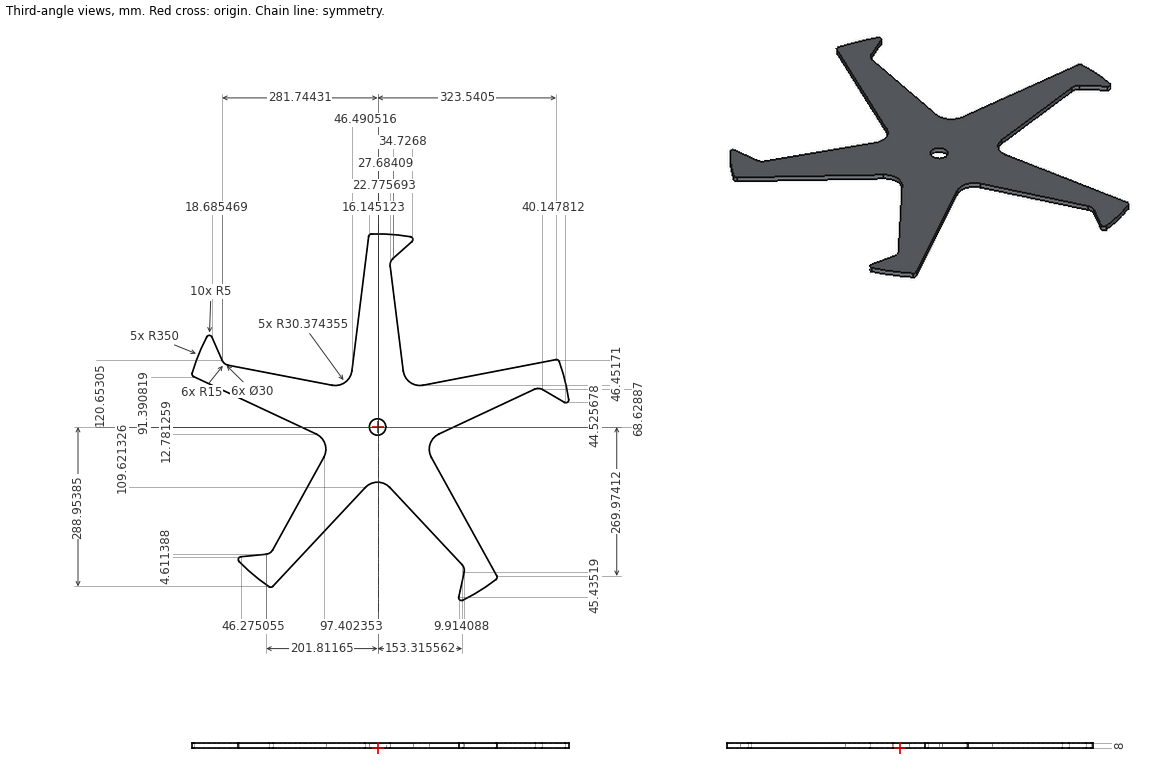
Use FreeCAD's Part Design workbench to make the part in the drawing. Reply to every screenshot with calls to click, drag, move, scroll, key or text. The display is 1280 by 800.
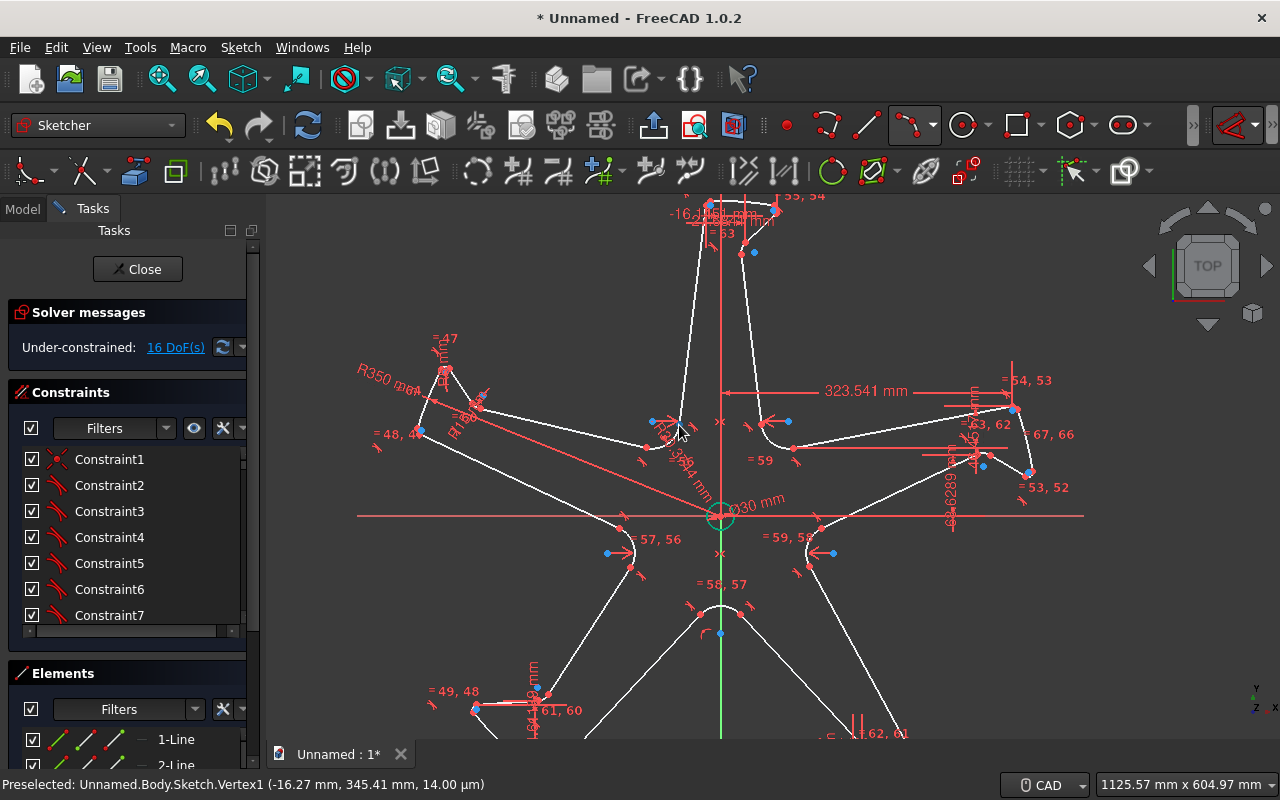
click(680, 425)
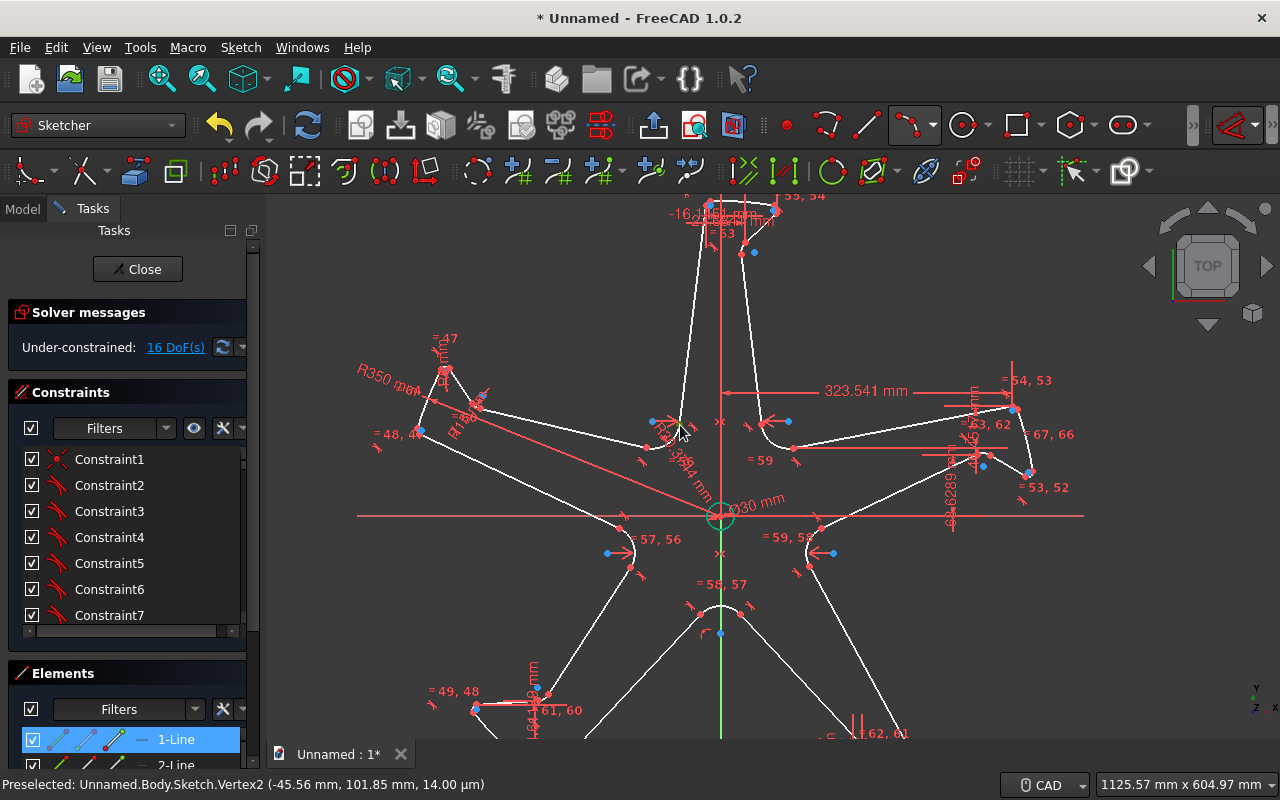
key(l)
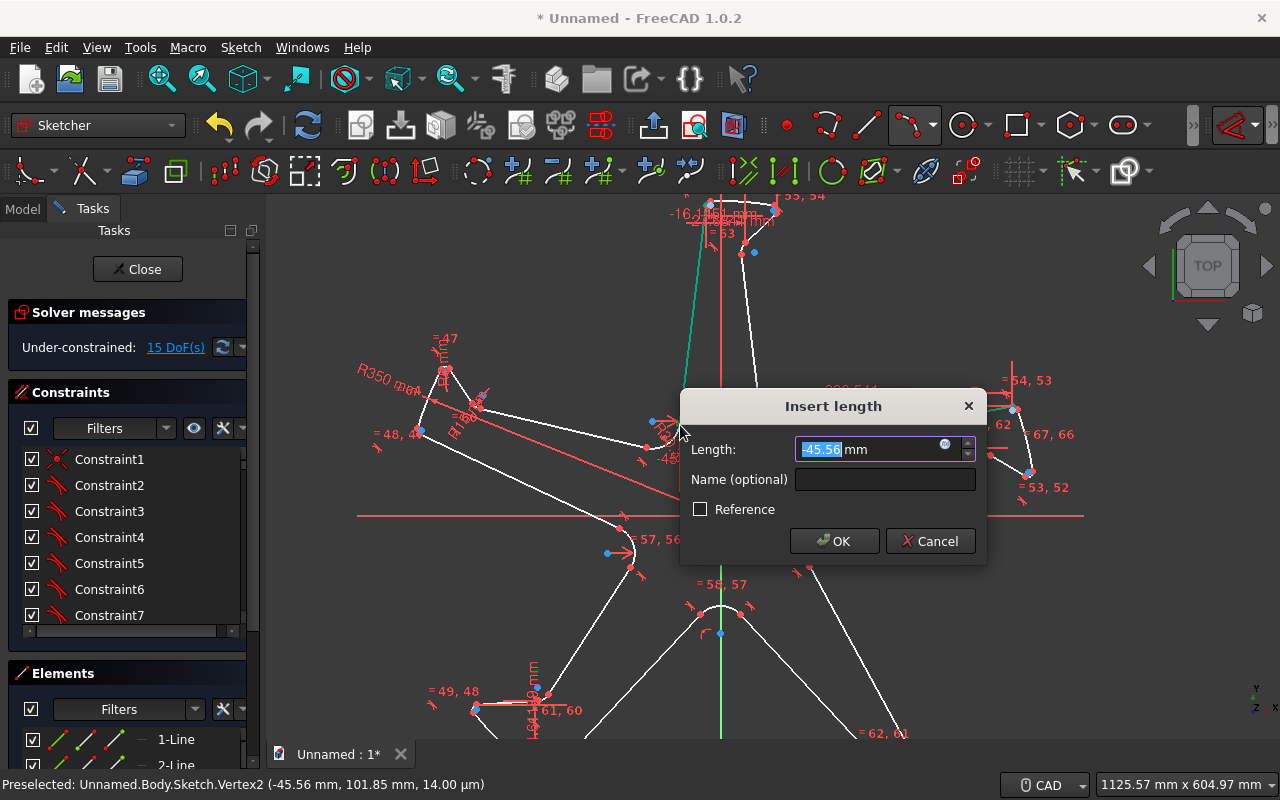
text(-46.490516)
key(Return)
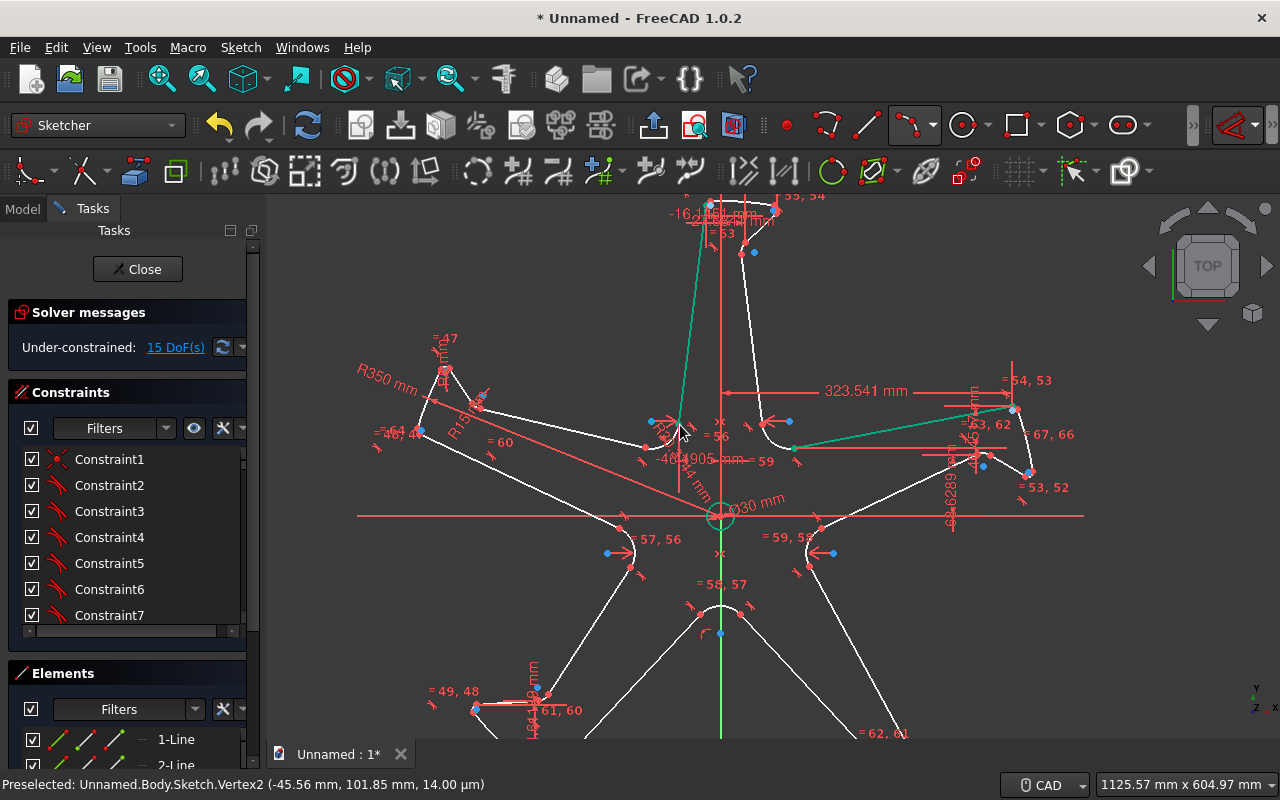
scroll(472, 403, up, 2)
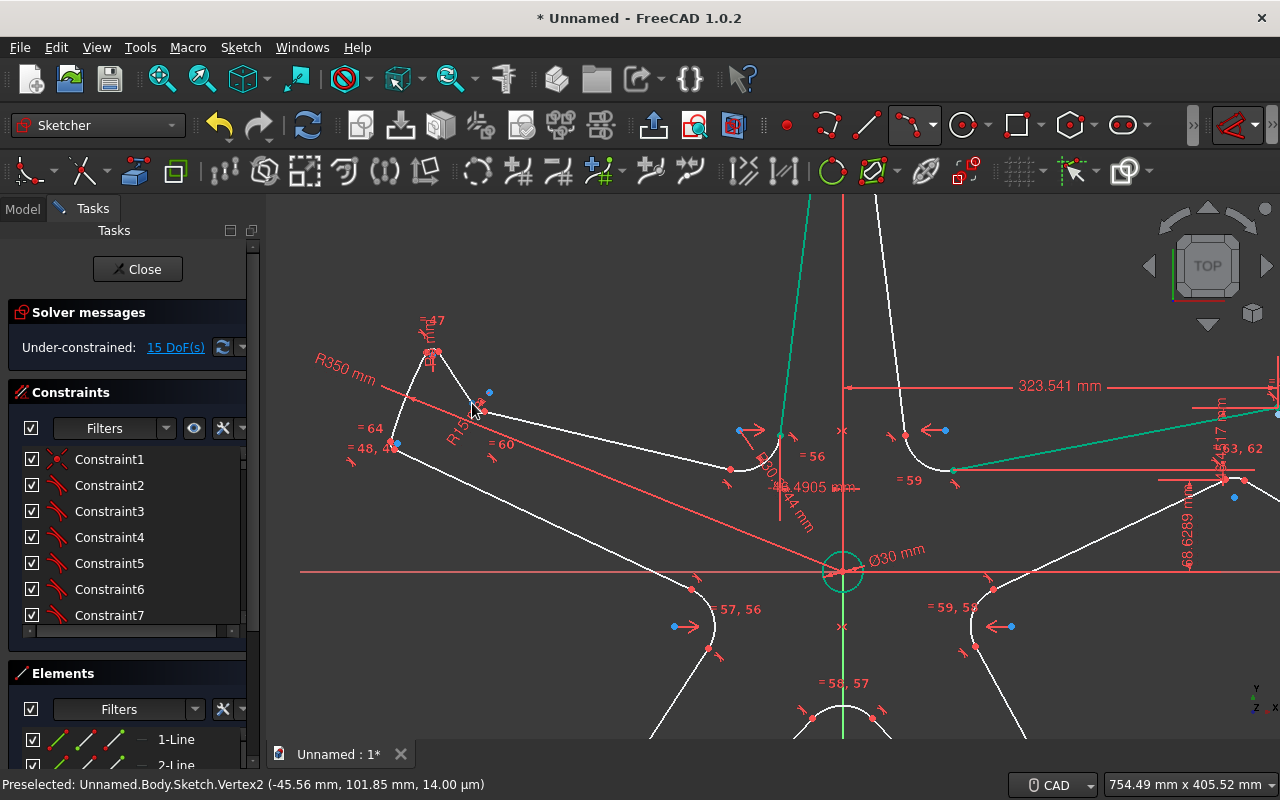
click(472, 403)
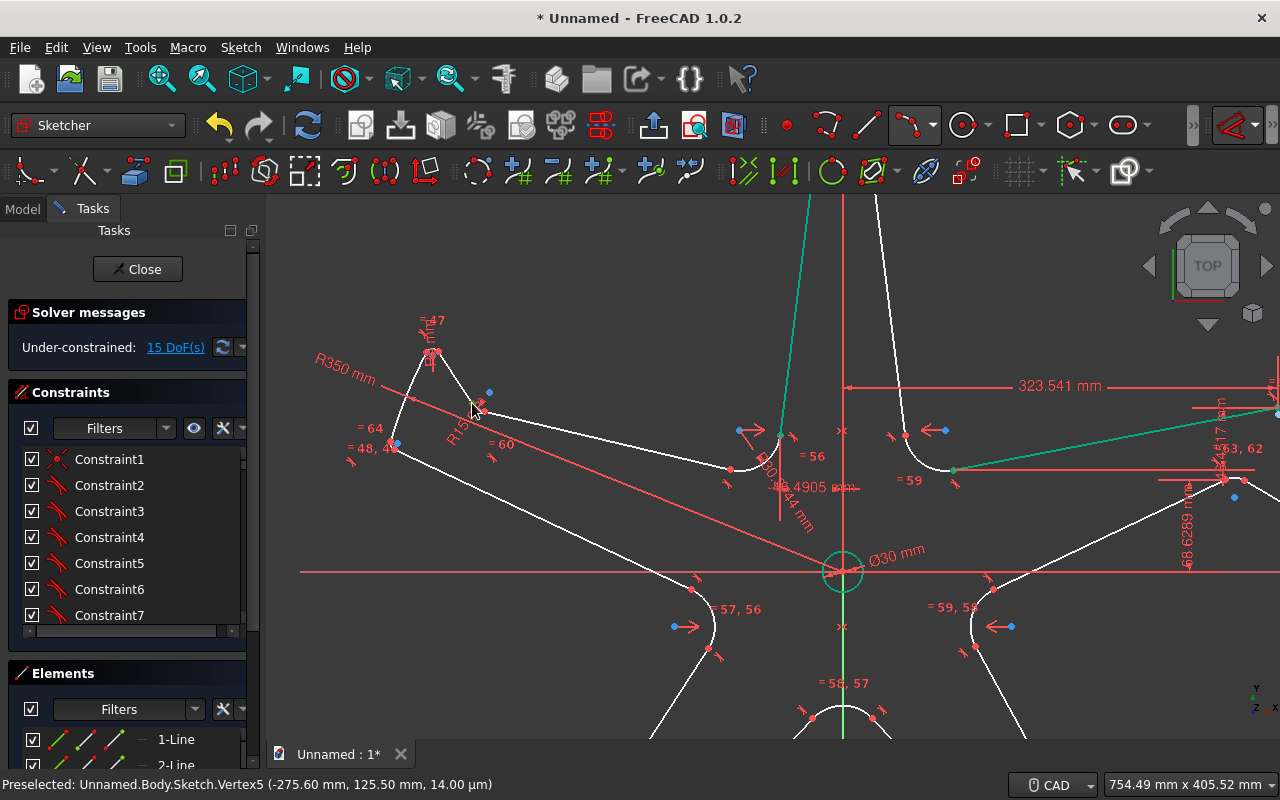
key(l)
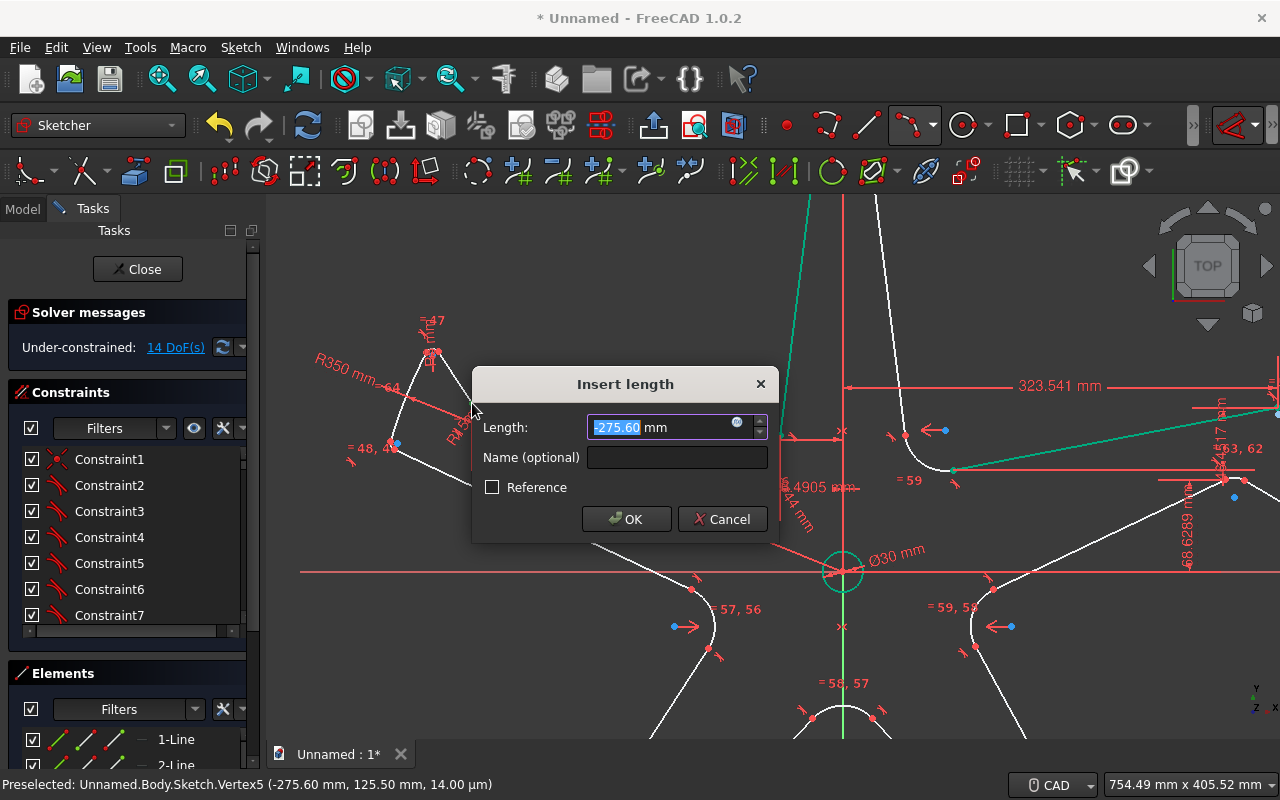
text(-281.74431)
key(Return)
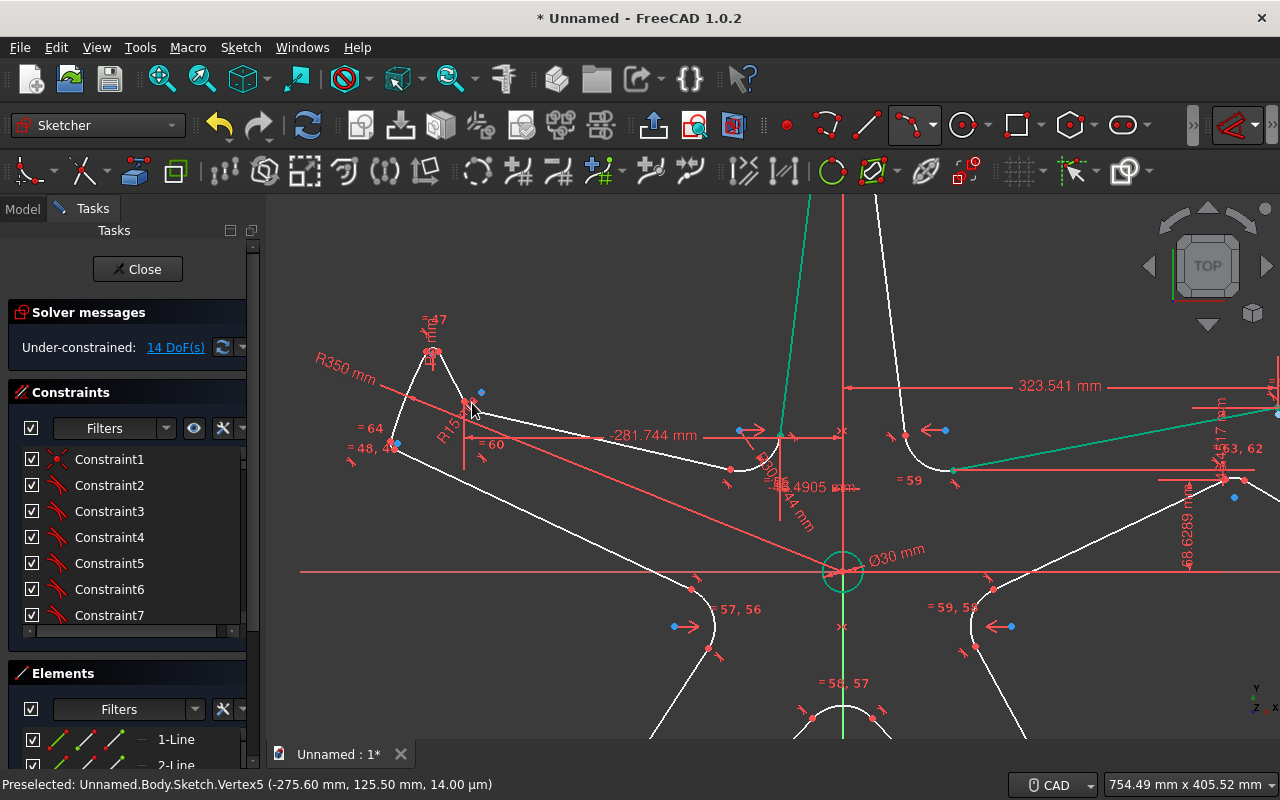
click(464, 401)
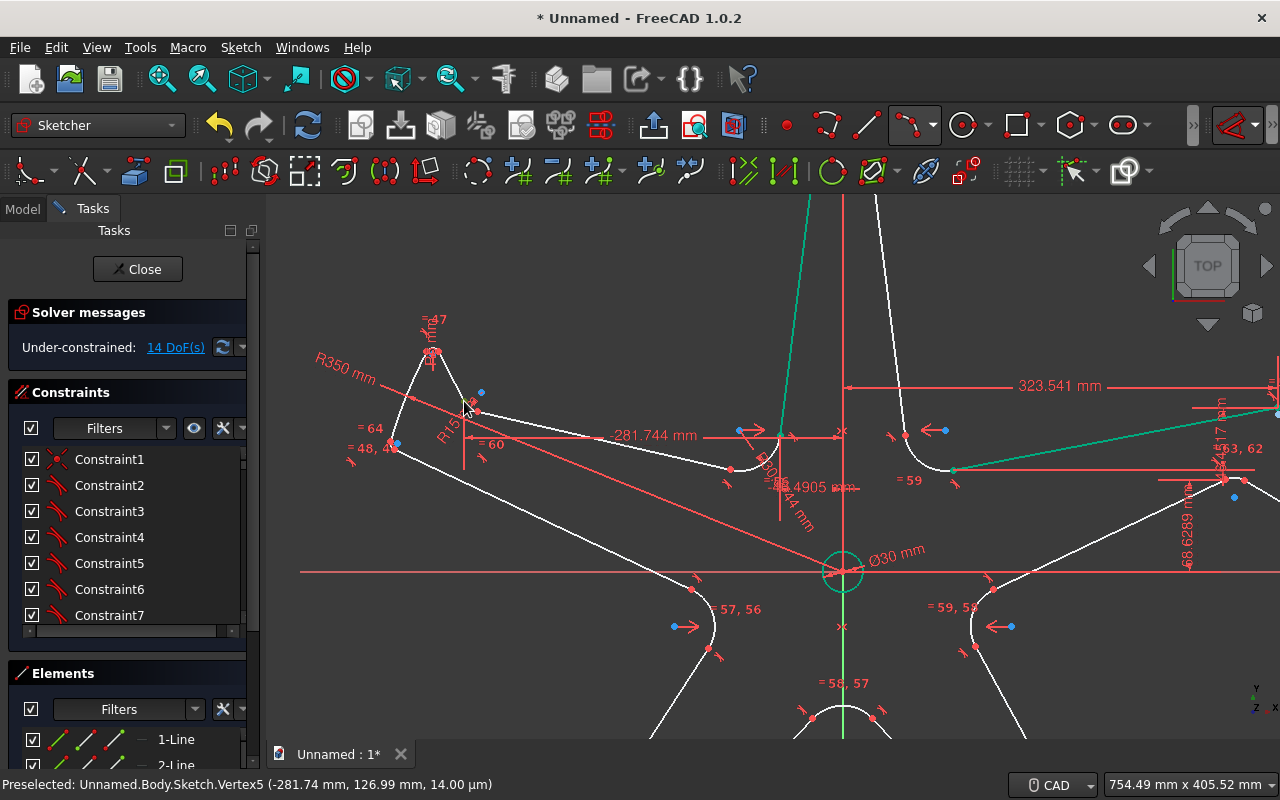
click(1258, 126)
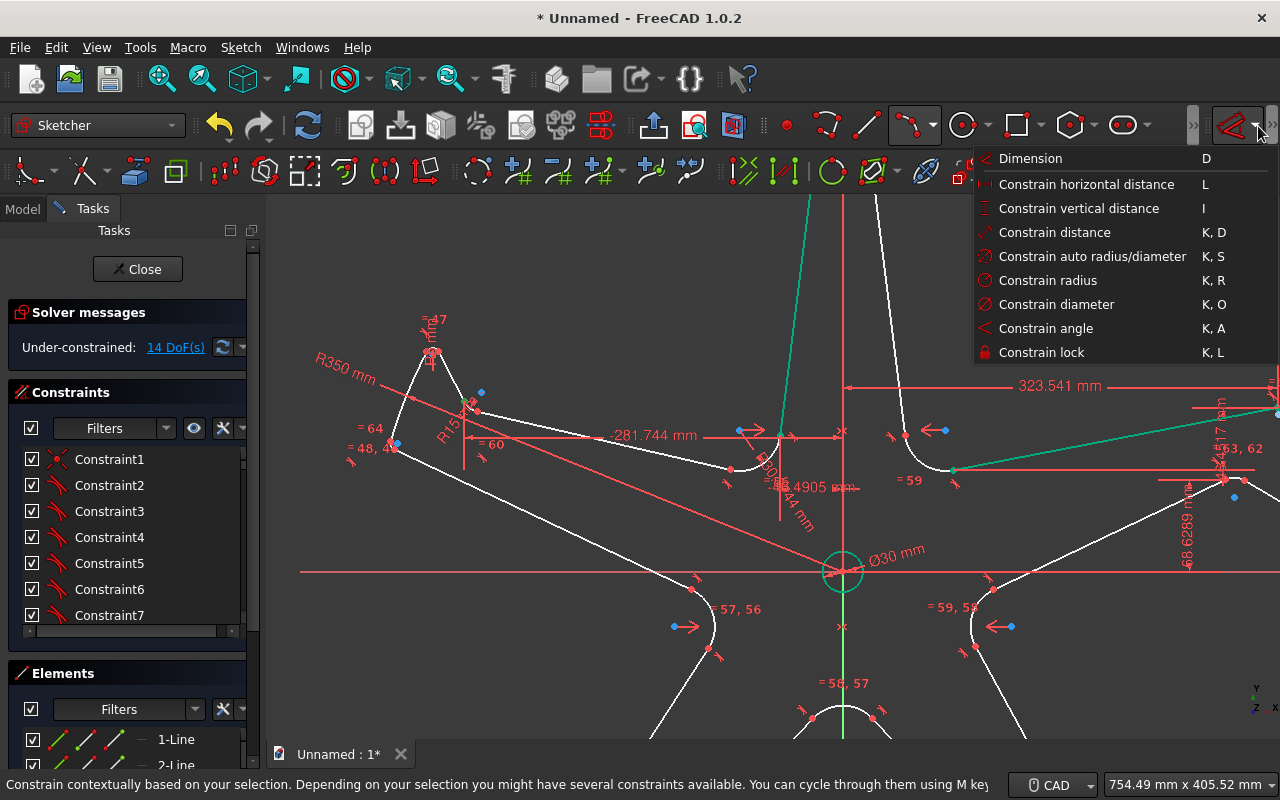
click(1126, 208)